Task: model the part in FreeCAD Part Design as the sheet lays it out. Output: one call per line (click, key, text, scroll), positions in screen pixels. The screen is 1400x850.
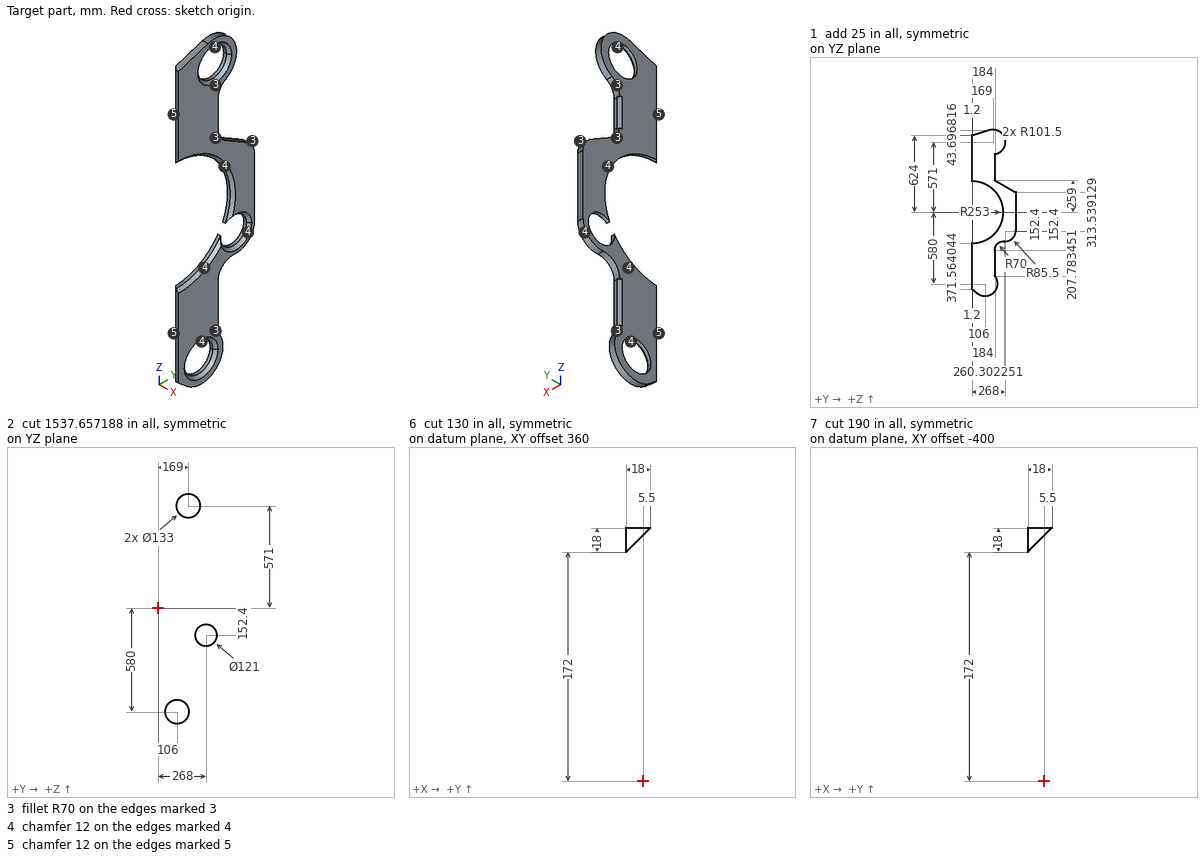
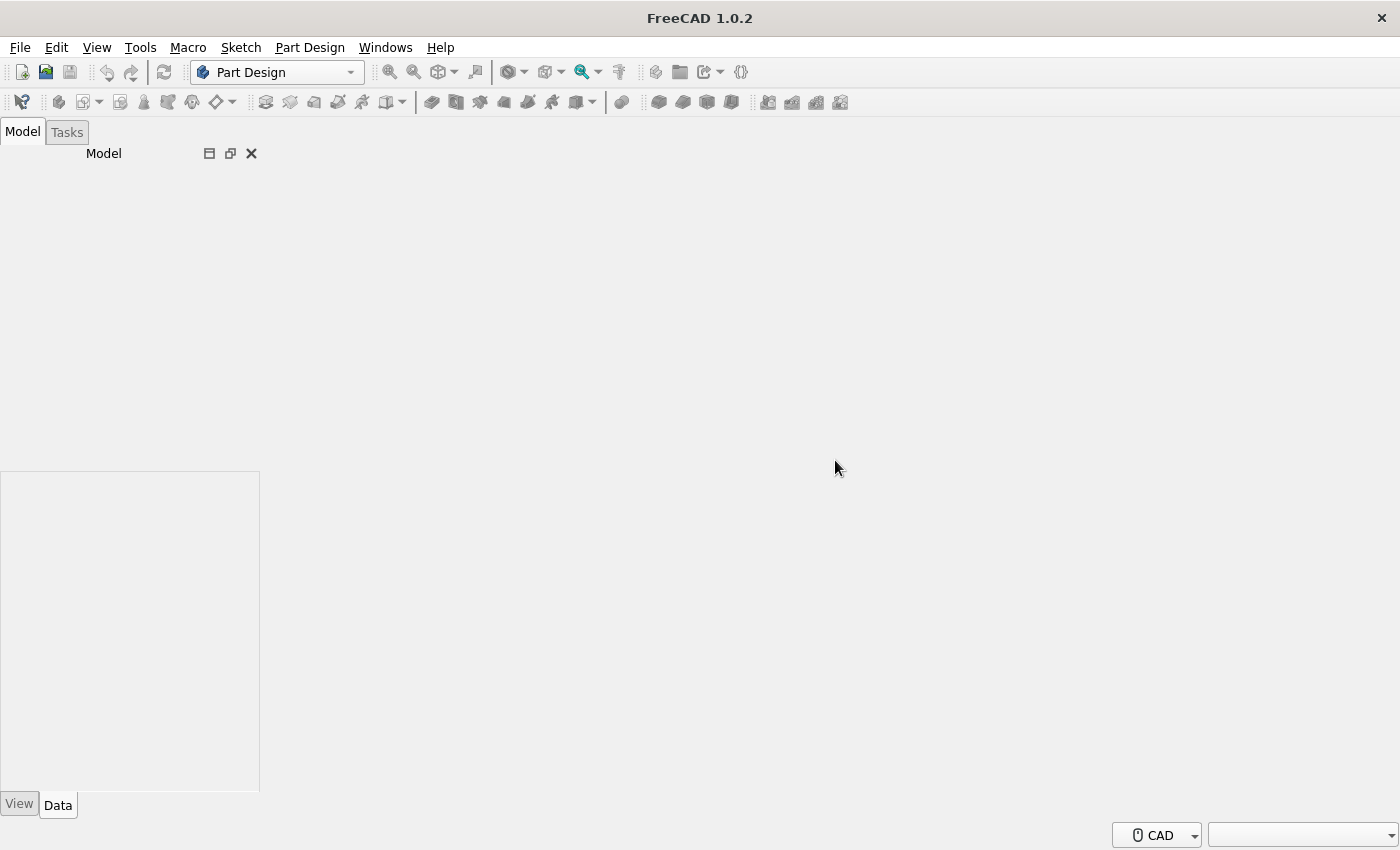
click(22, 72)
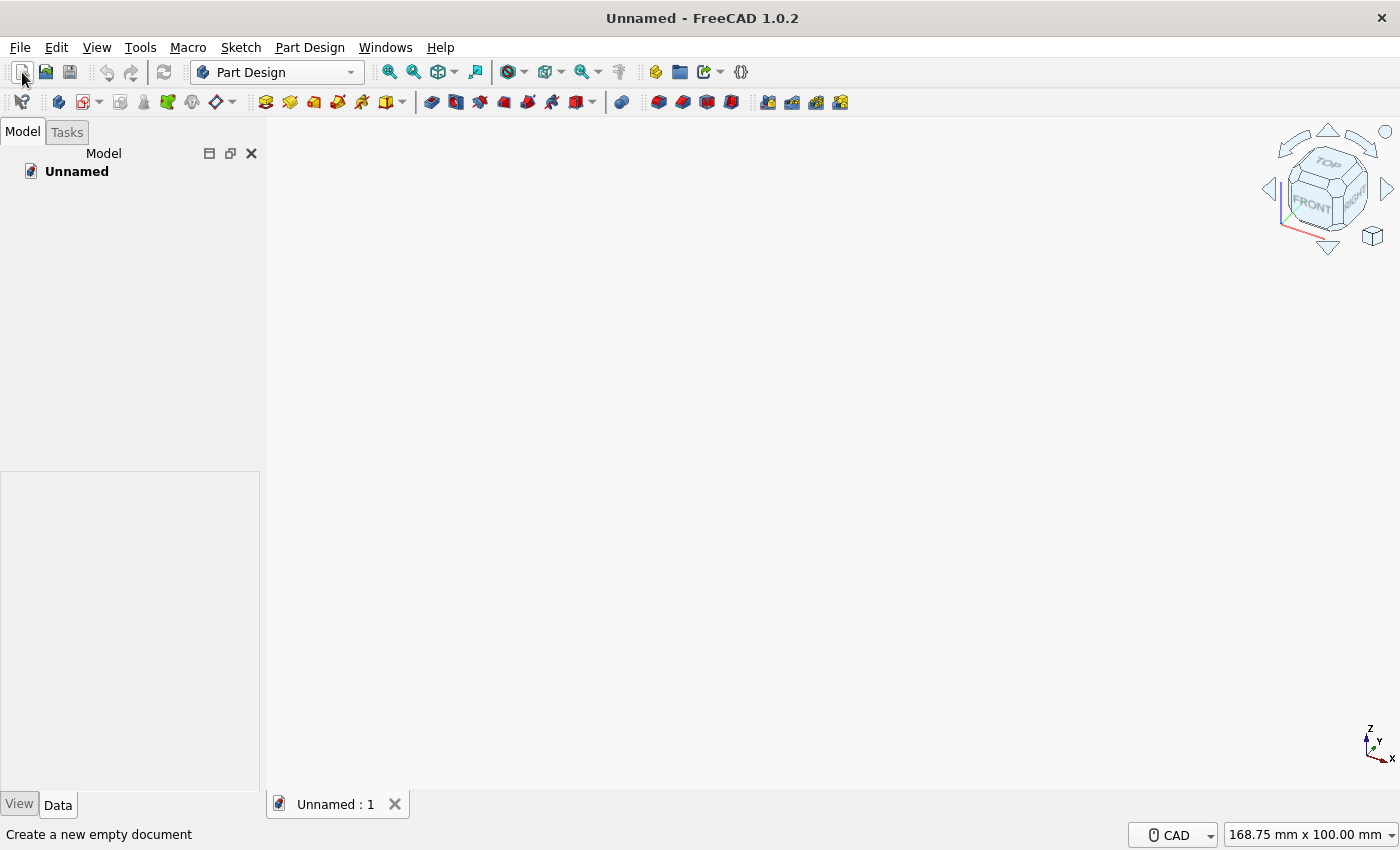
click(84, 102)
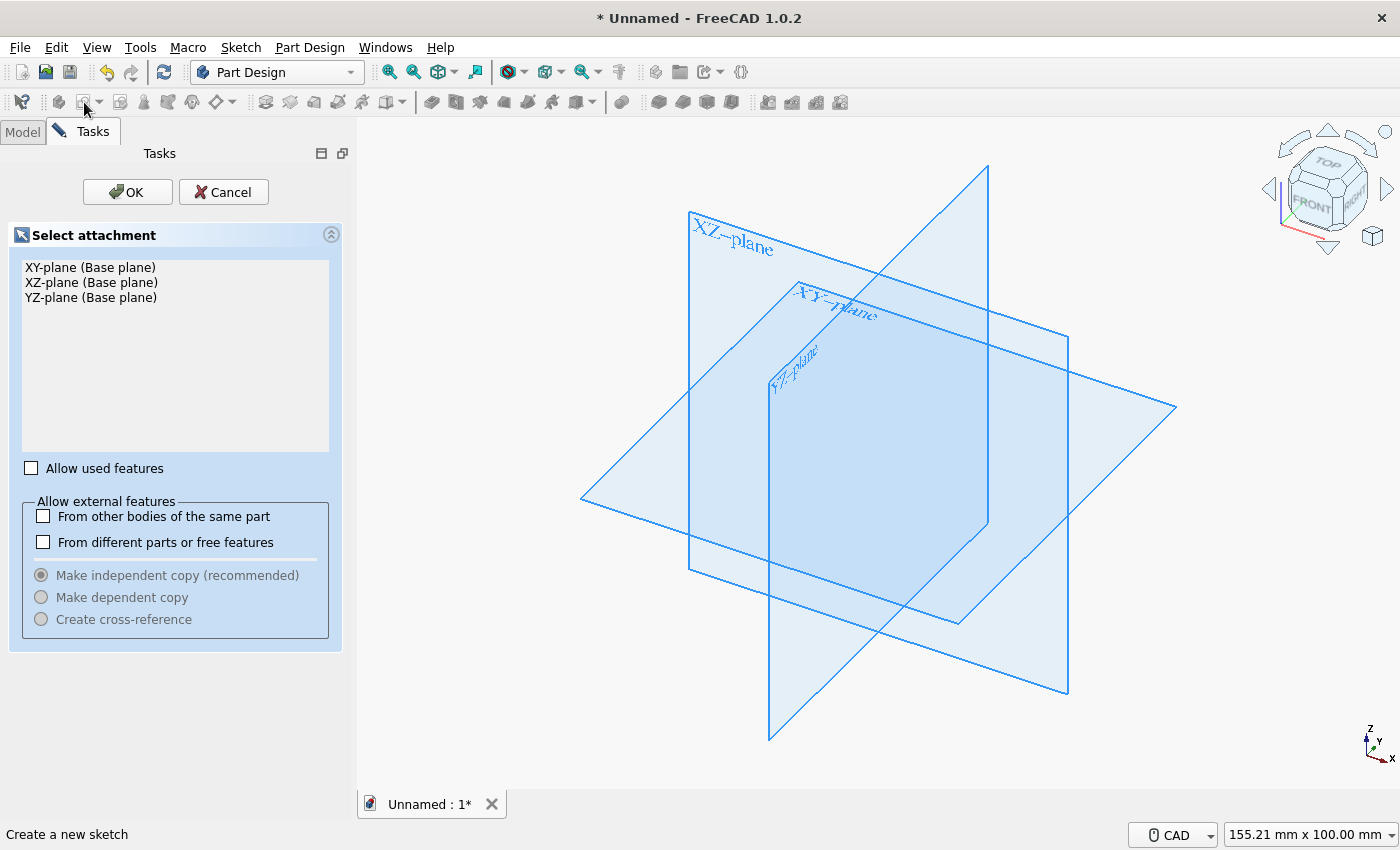
click(82, 298)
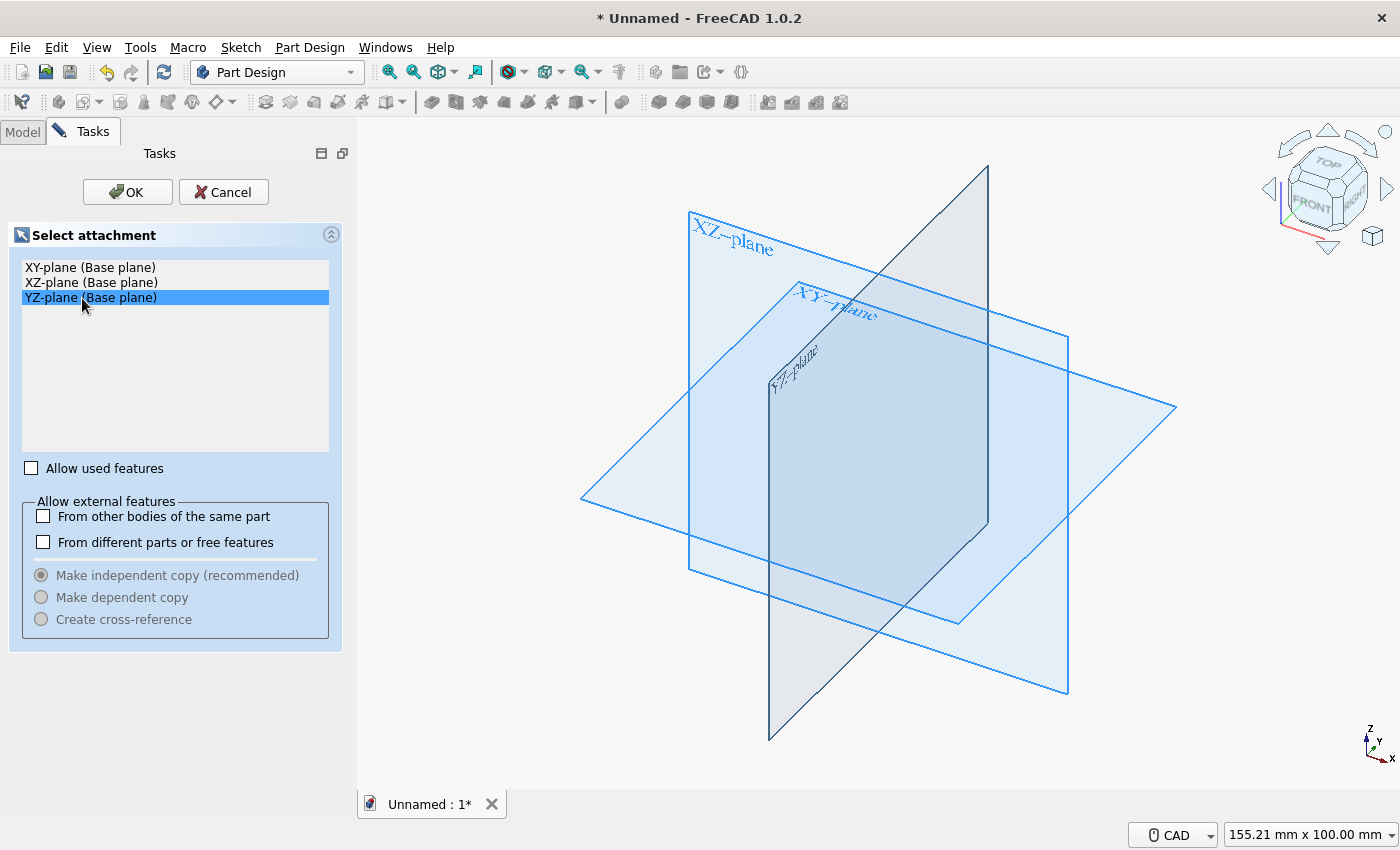
click(128, 192)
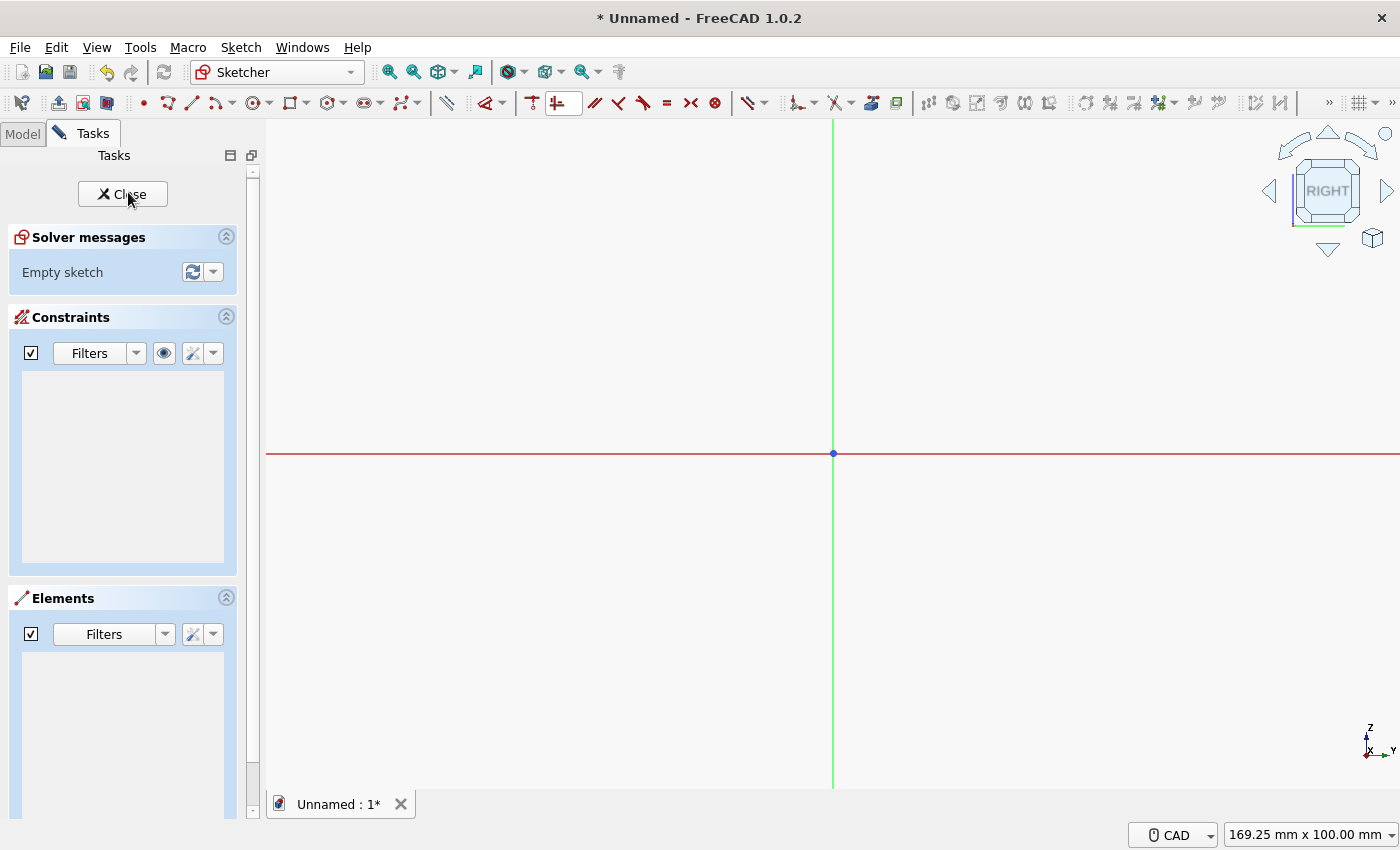
scroll(699, 456, down, 15)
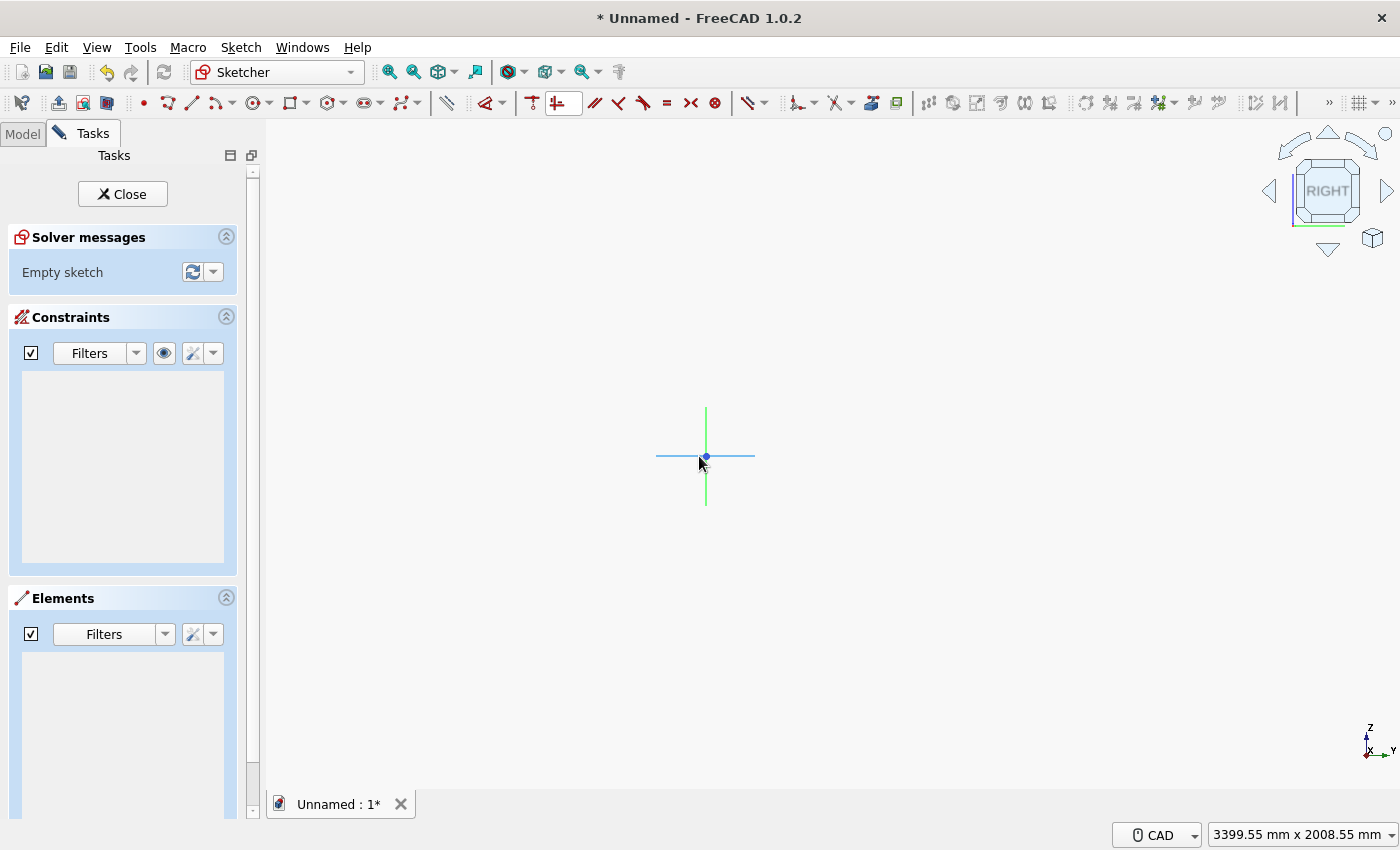
key(g)
key(m)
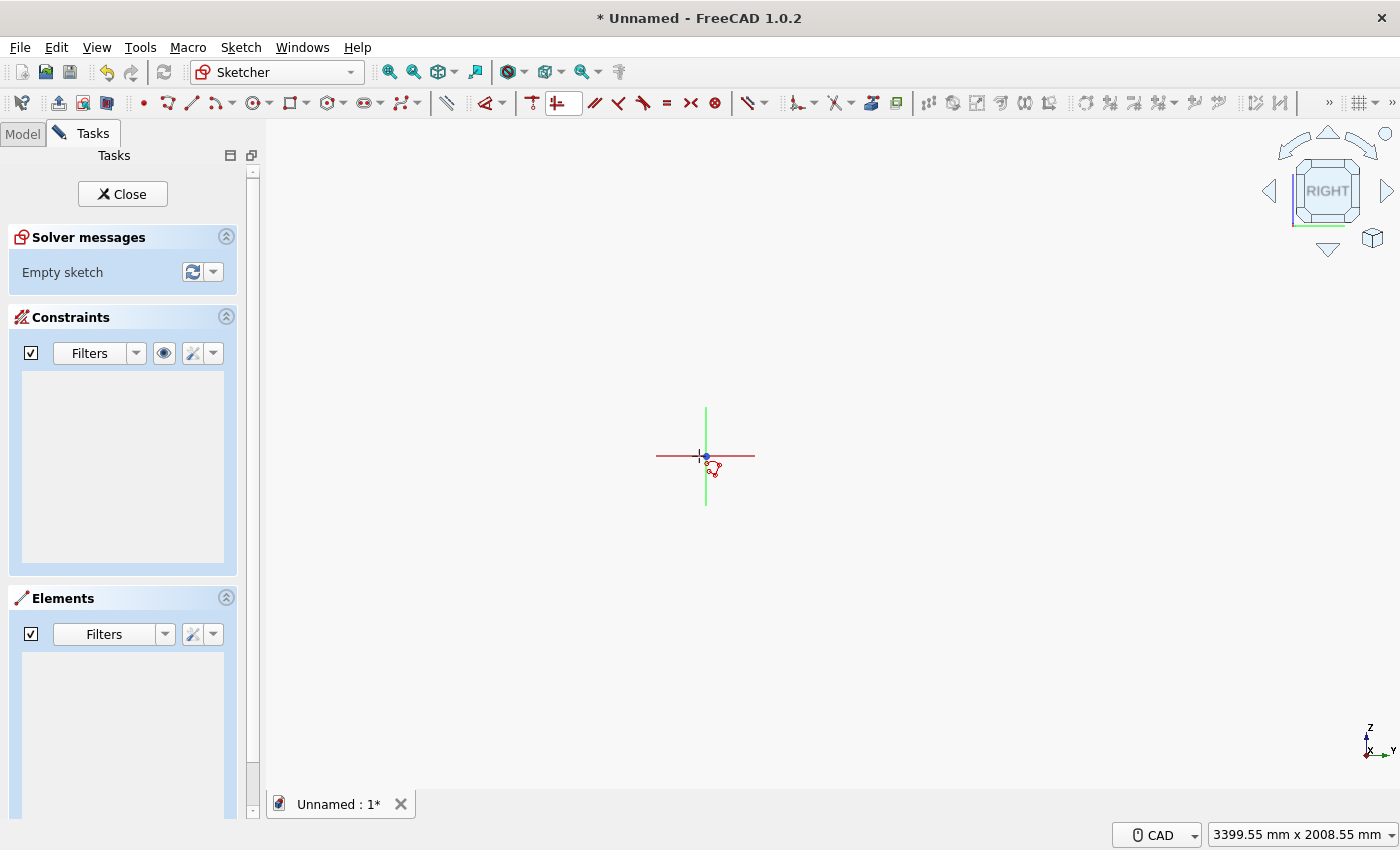
click(824, 507)
click(824, 403)
click(767, 370)
click(767, 299)
right_click(767, 299)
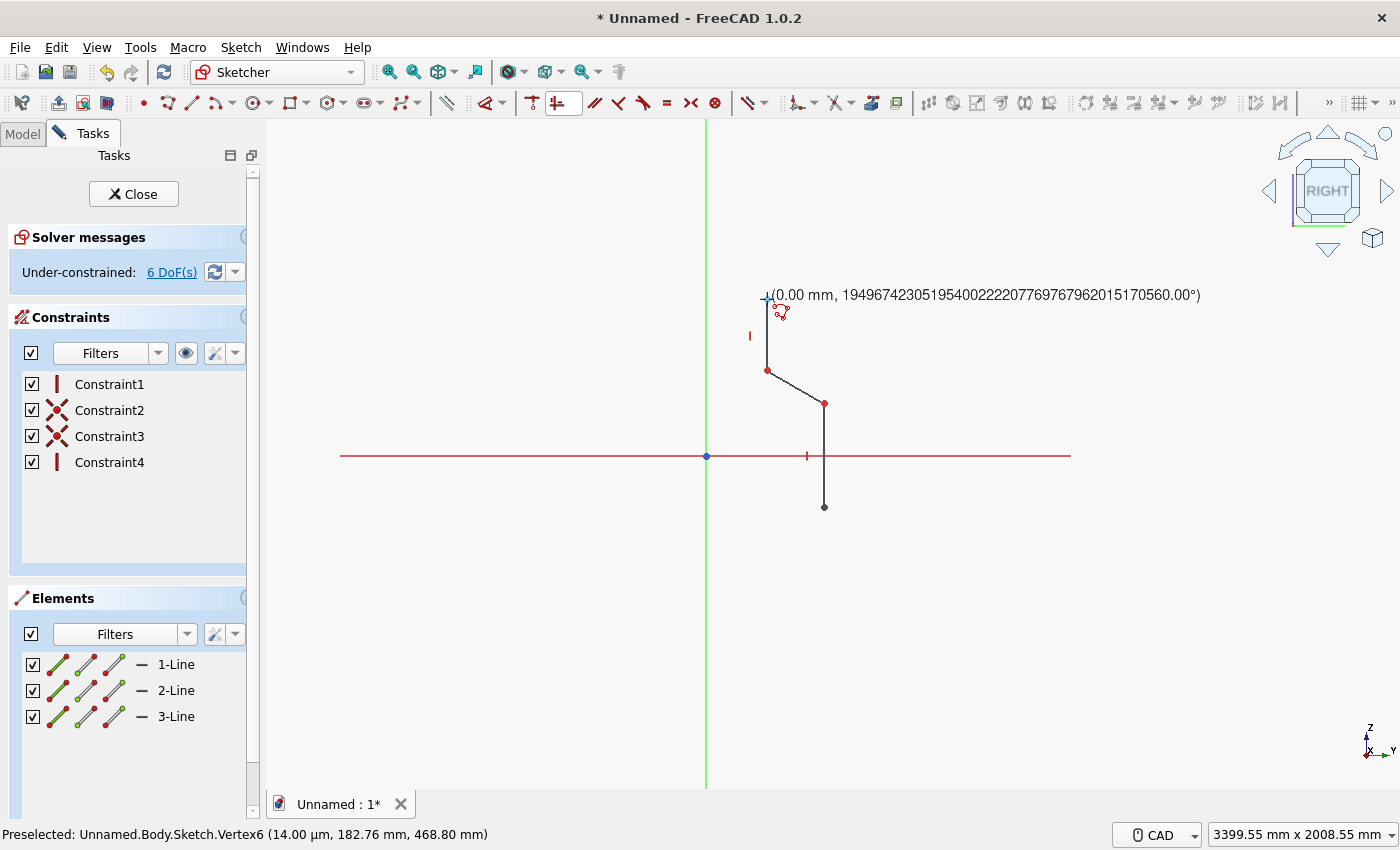
click(752, 234)